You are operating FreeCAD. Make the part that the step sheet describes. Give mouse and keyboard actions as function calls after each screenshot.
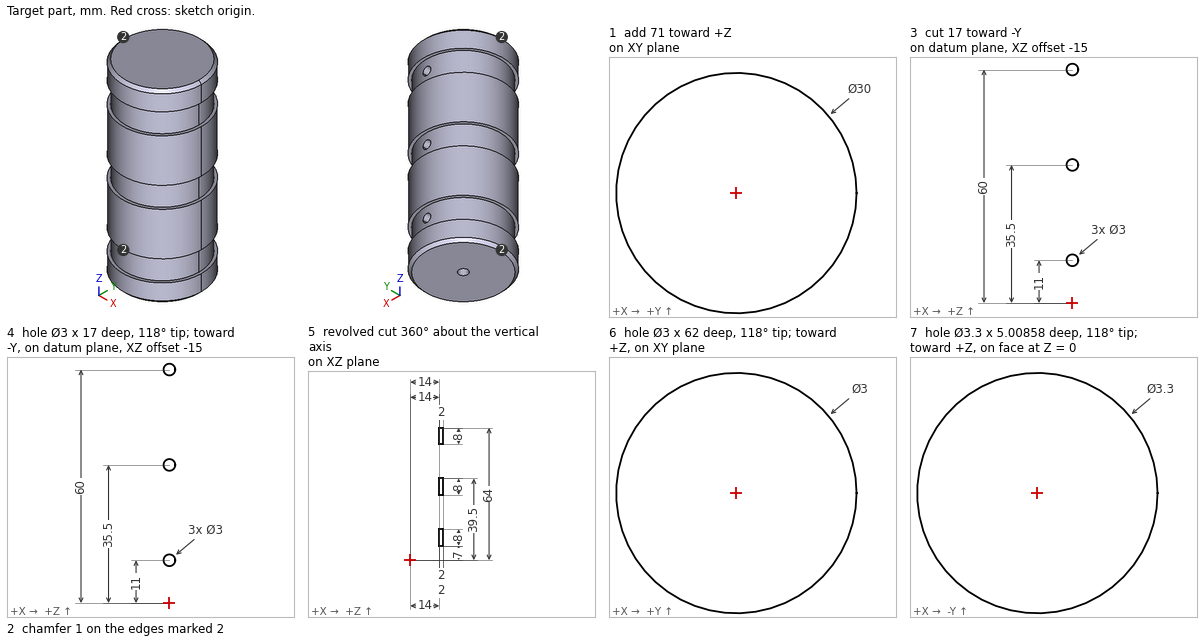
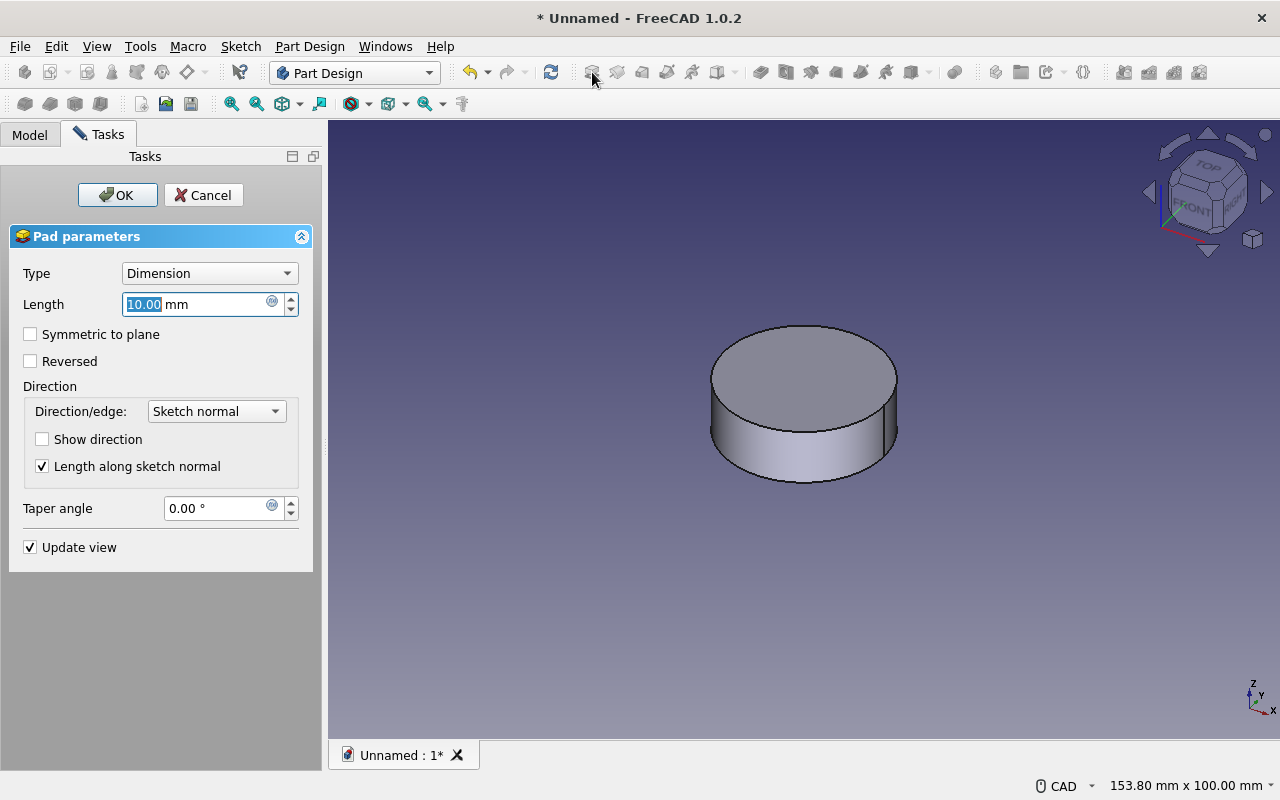
text(71)
key(Tab)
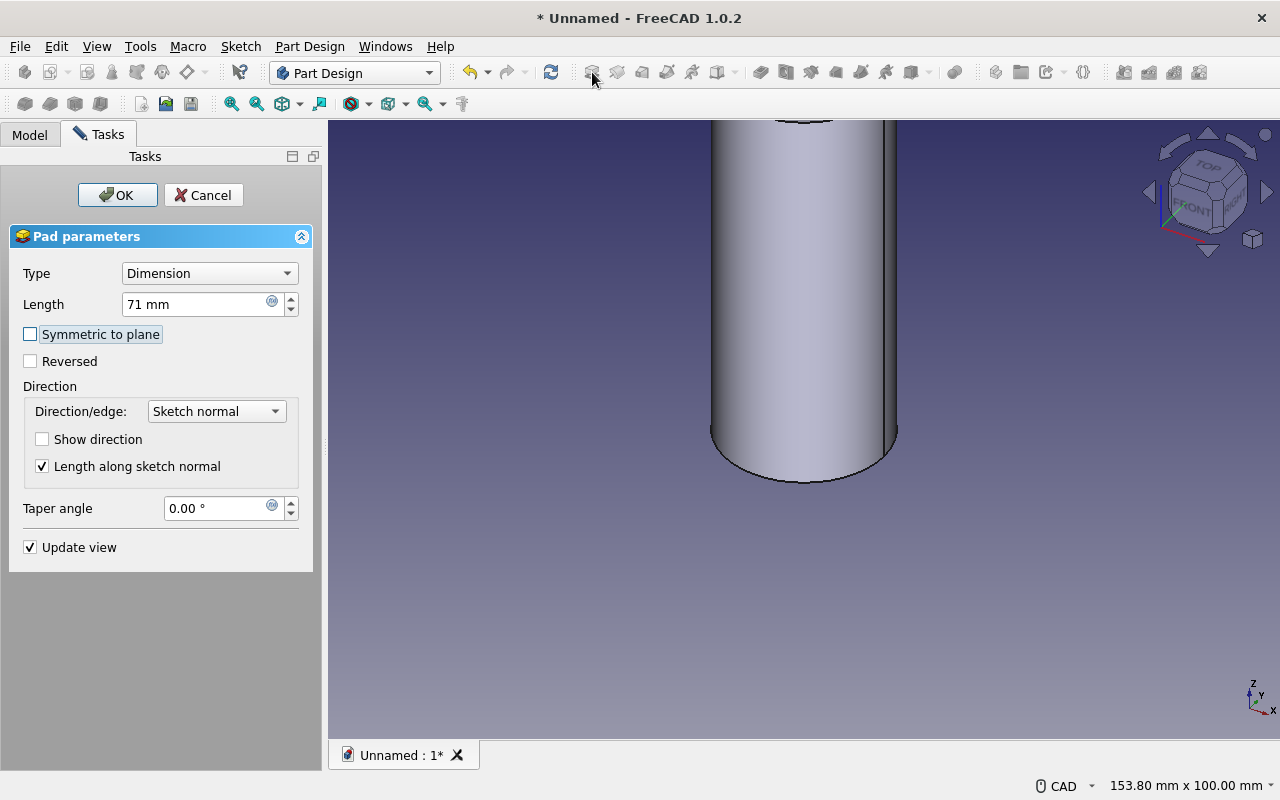
click(118, 195)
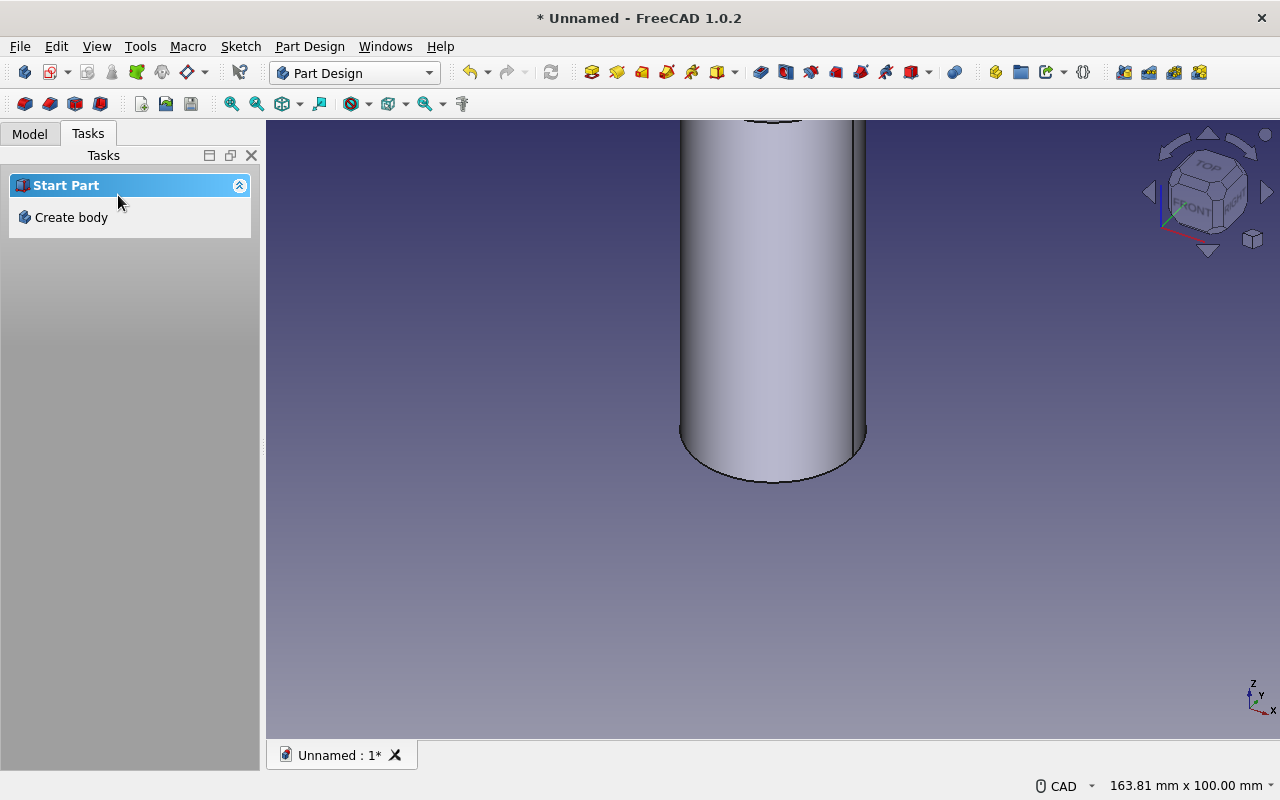
click(232, 104)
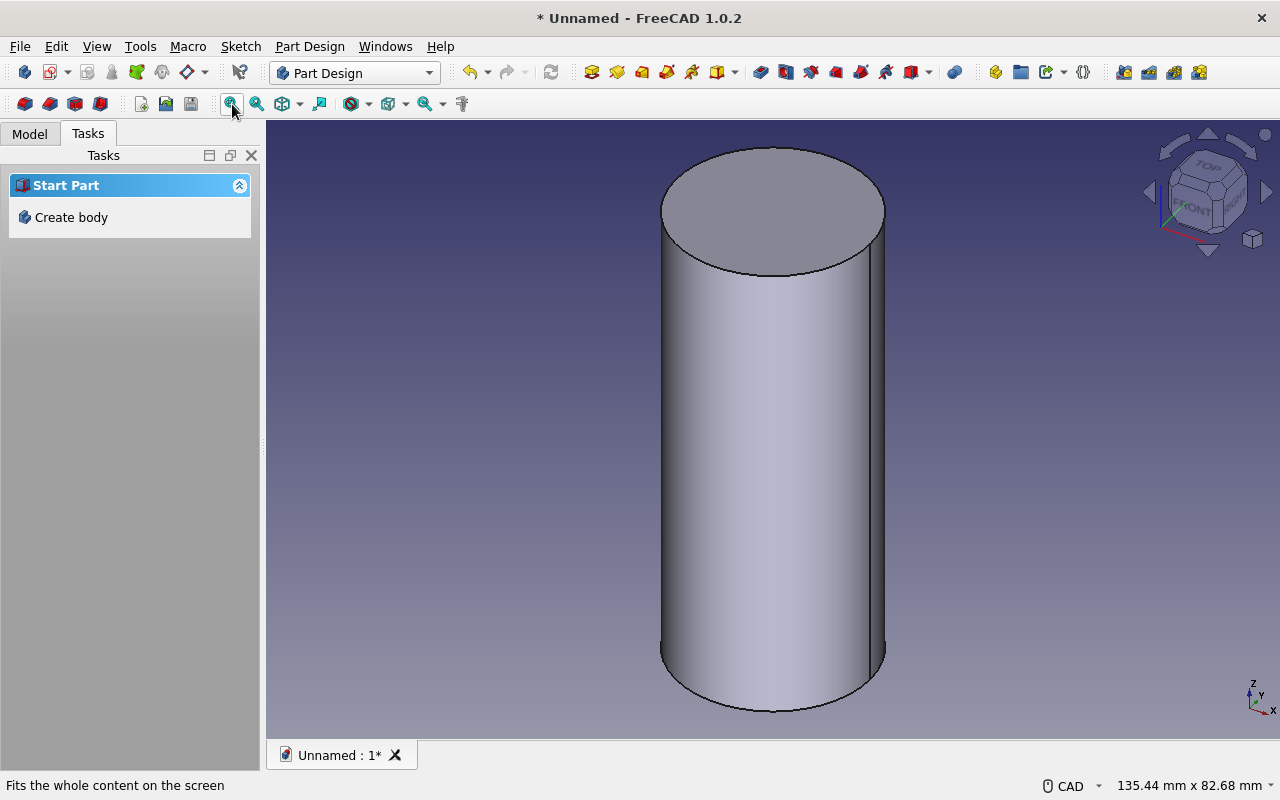
click(661, 218)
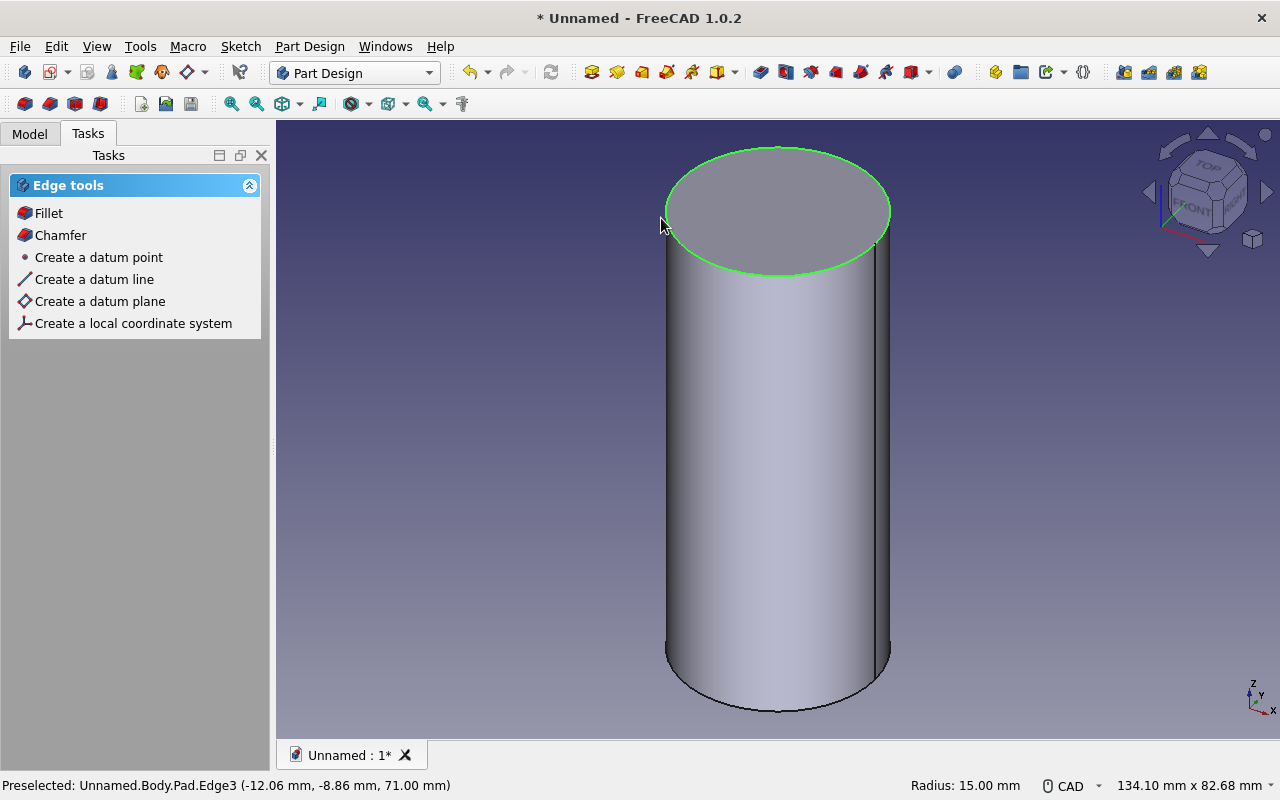
key(0)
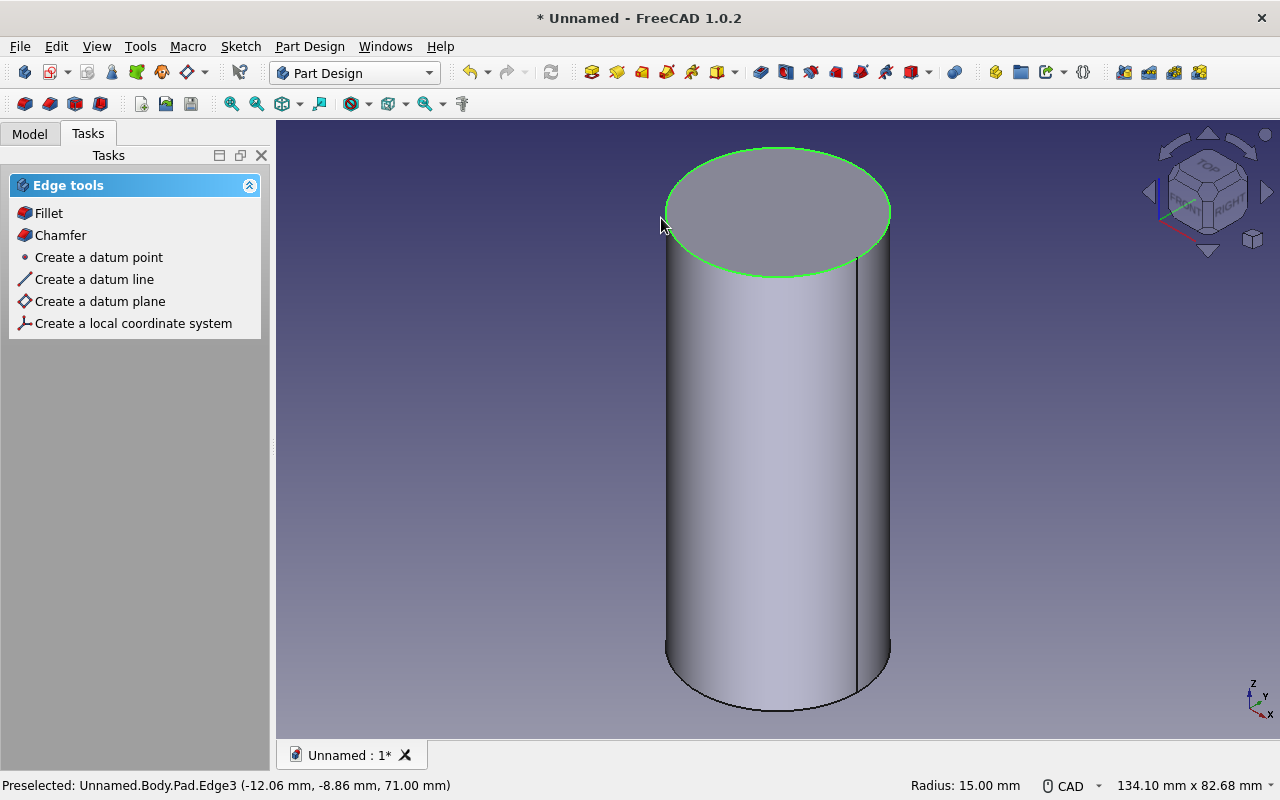
click(871, 682, ctrl)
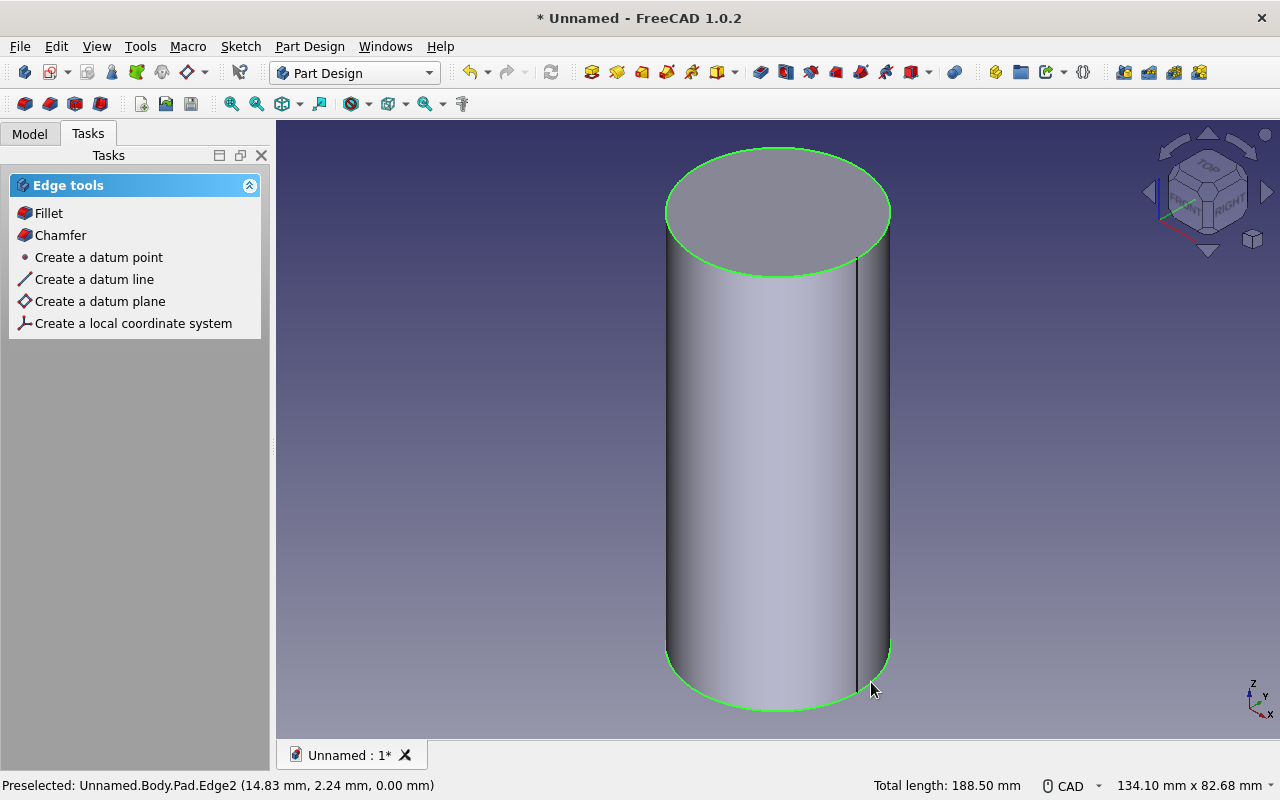
click(50, 104)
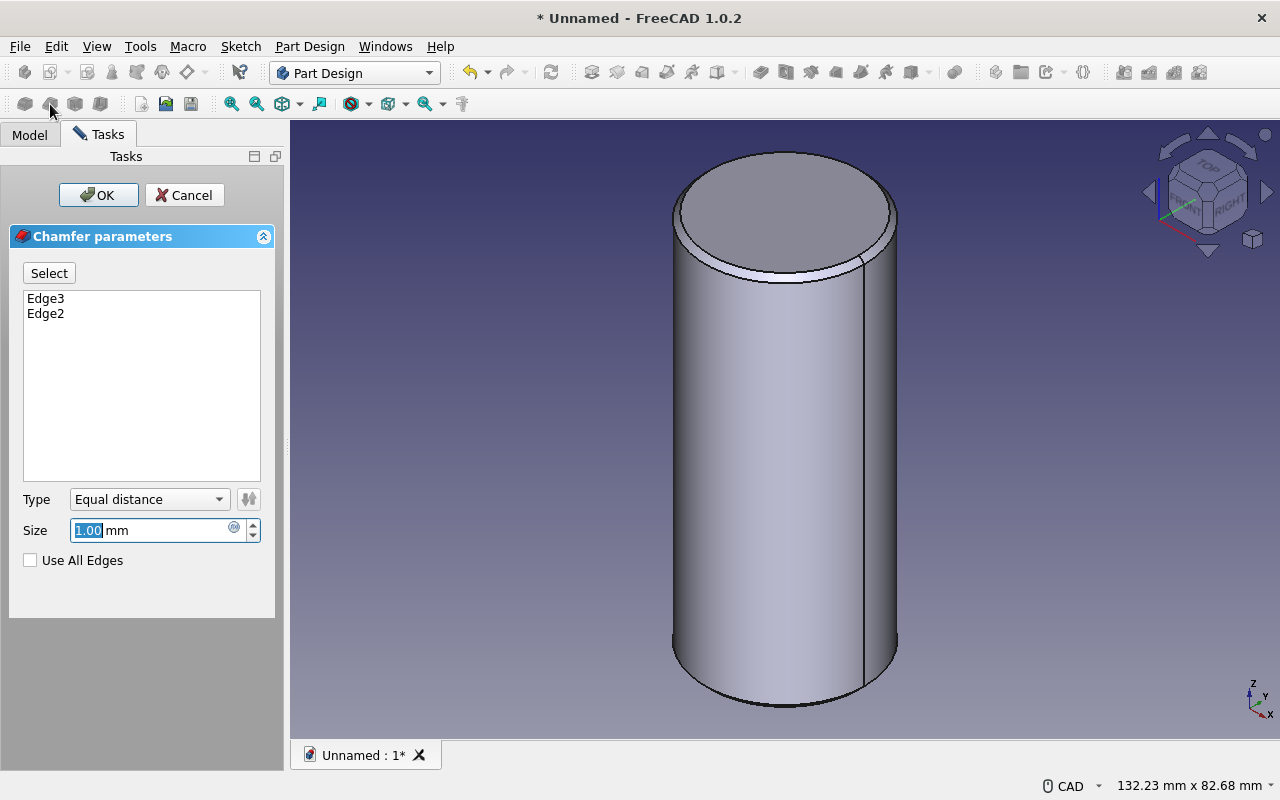
text(1)
key(Tab)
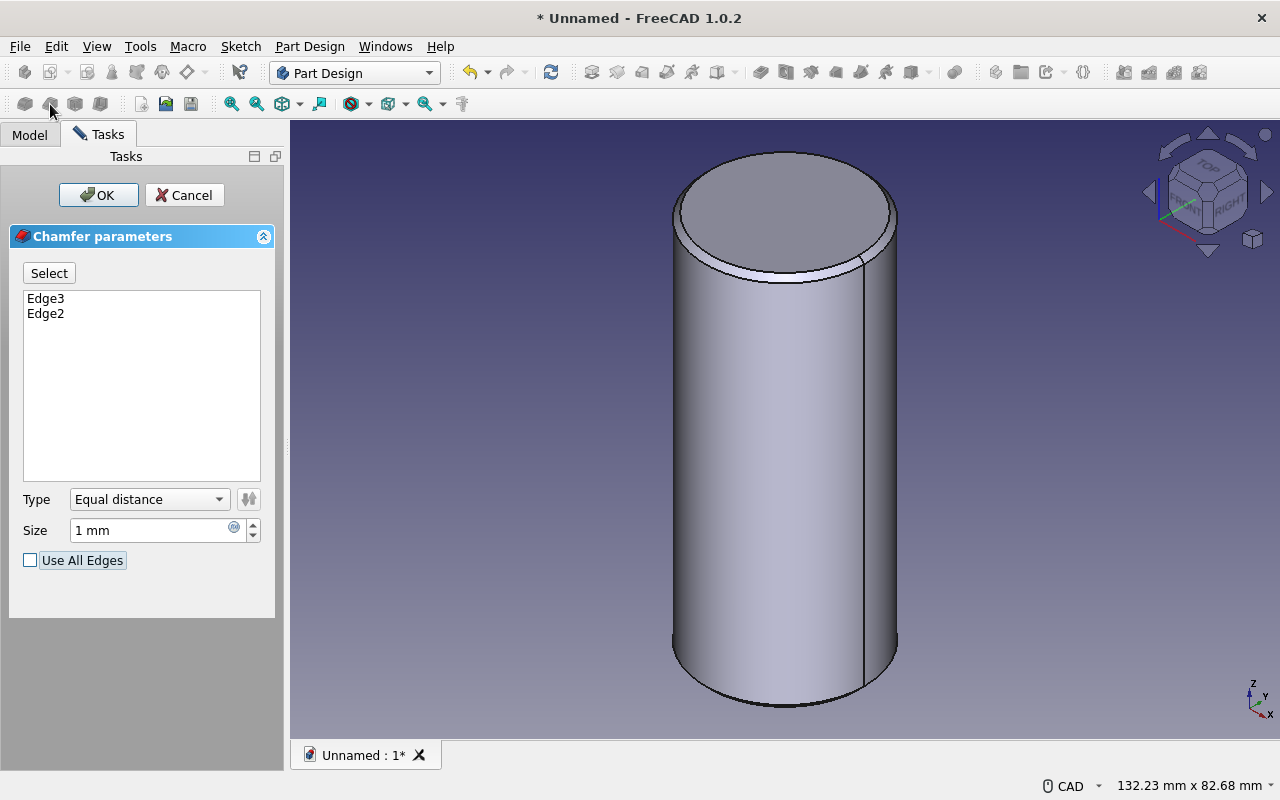
click(99, 195)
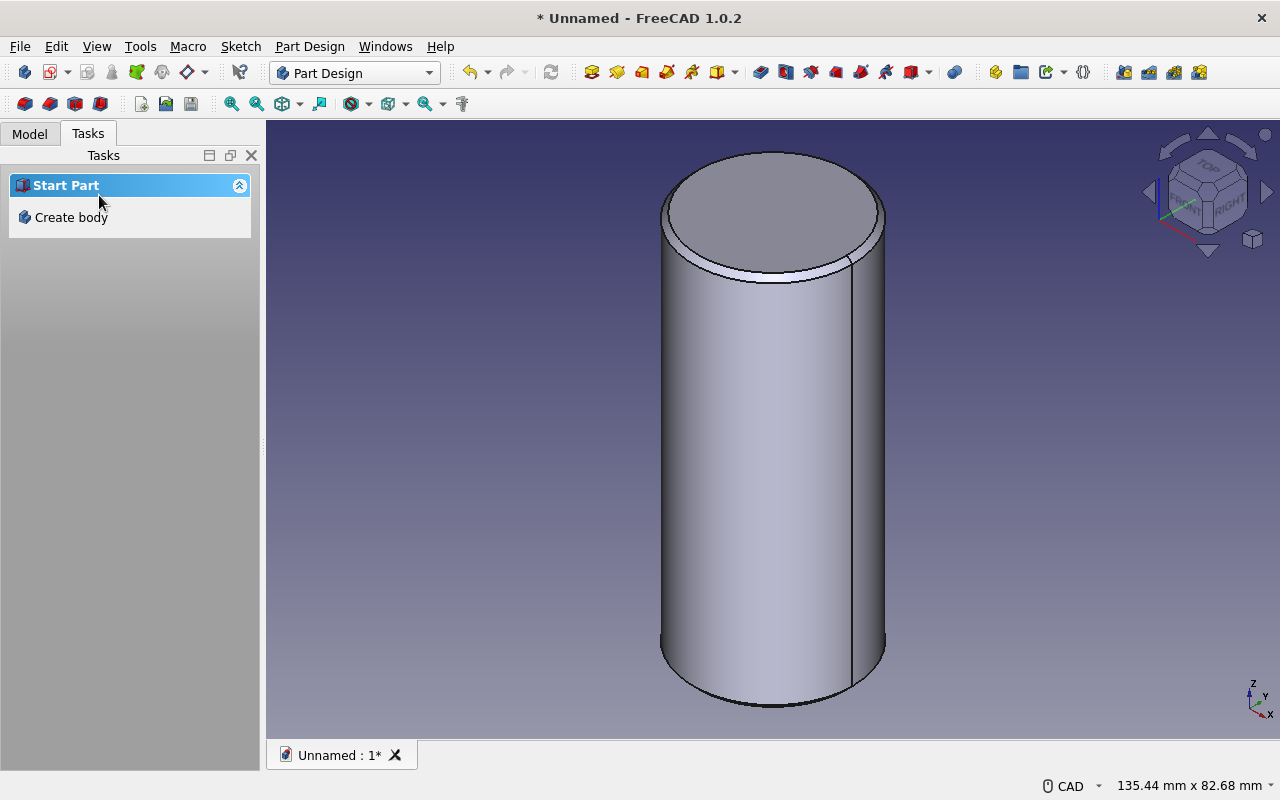
click(30, 134)